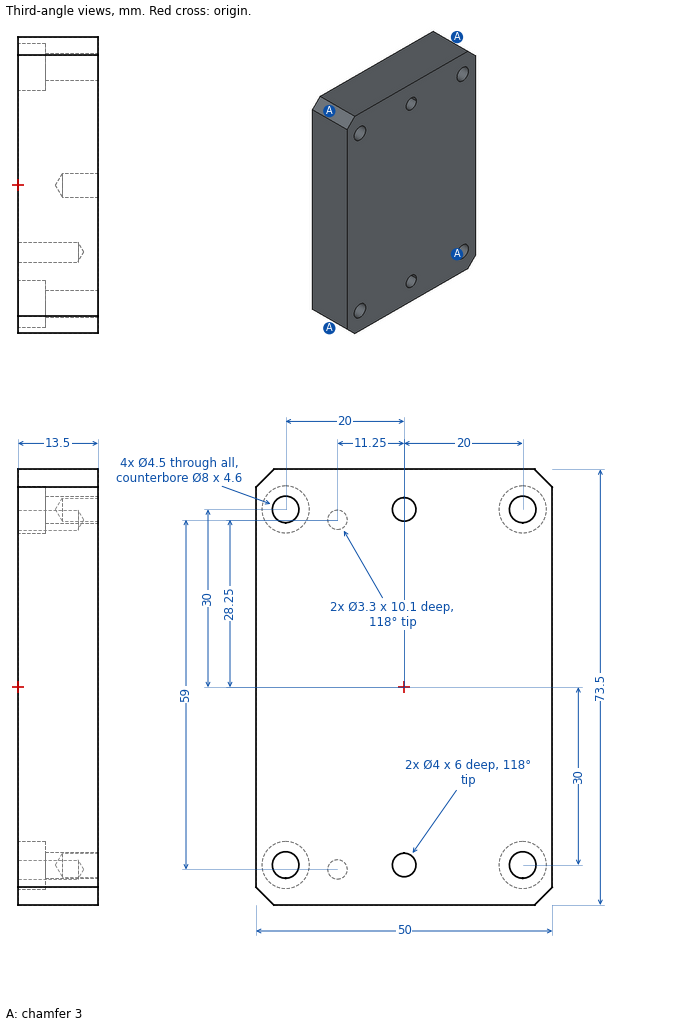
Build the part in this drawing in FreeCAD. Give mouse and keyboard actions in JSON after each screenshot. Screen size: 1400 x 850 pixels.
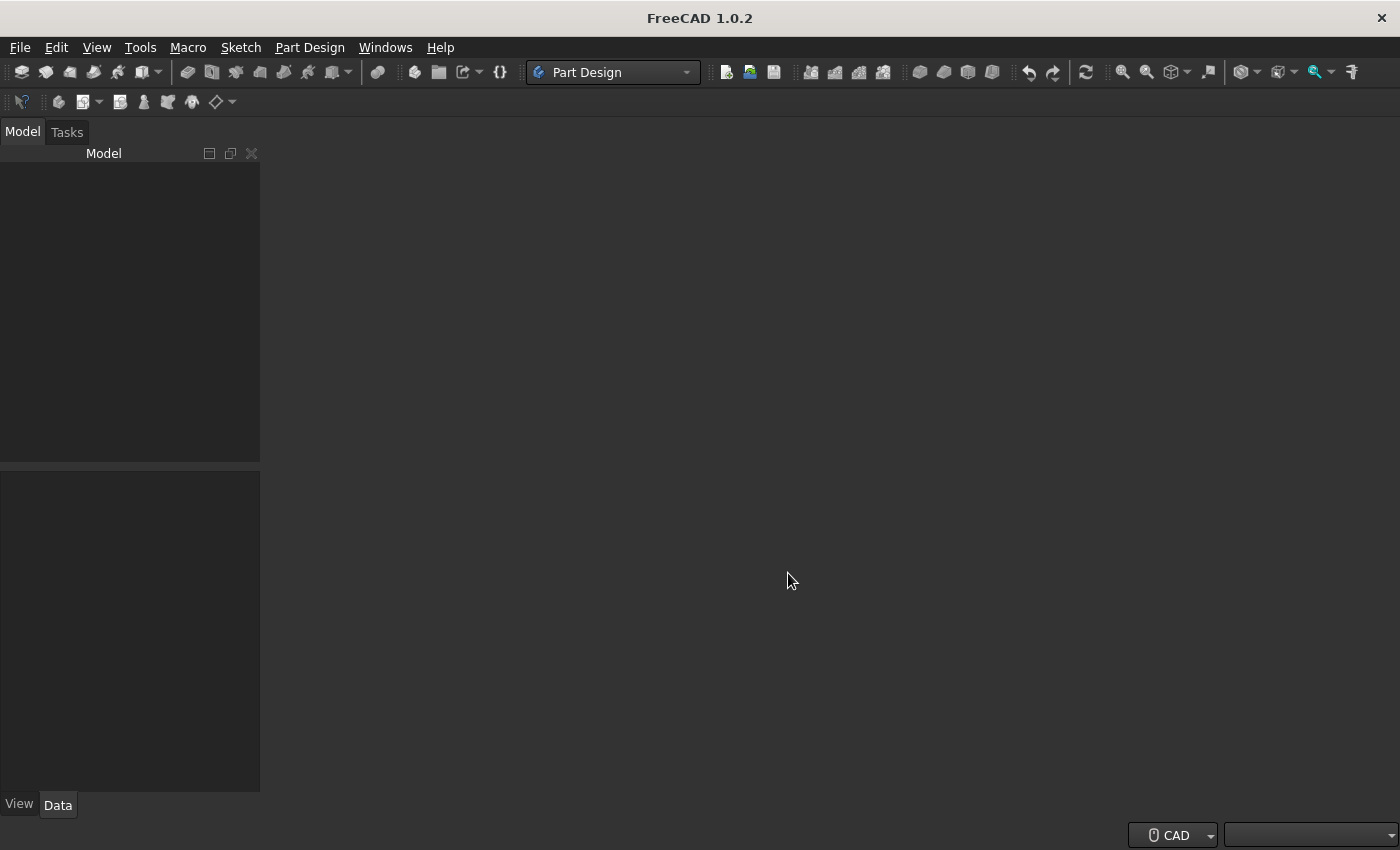
{"action": "left_click", "coordinate": [726, 72]}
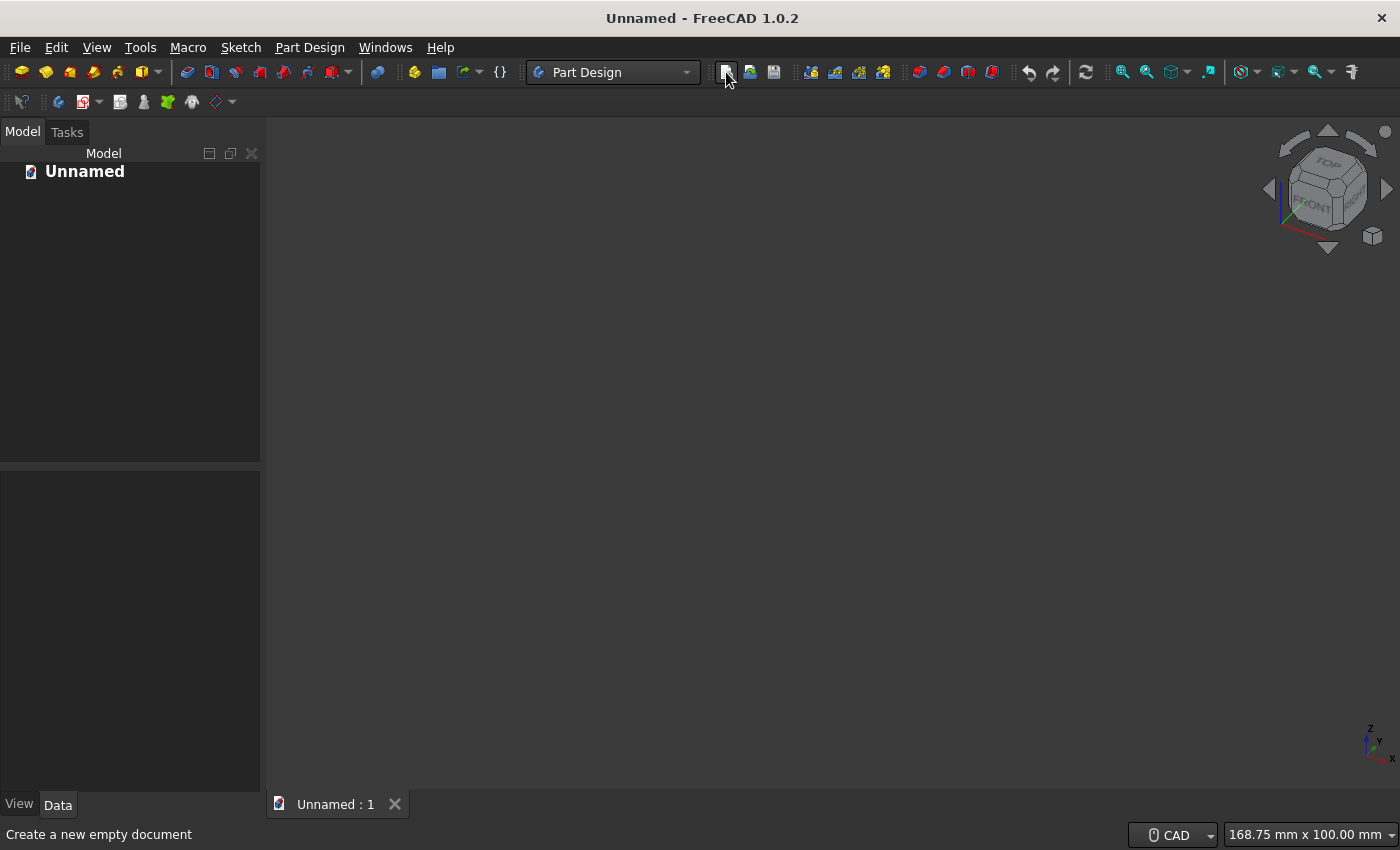
{"action": "left_click", "coordinate": [84, 102]}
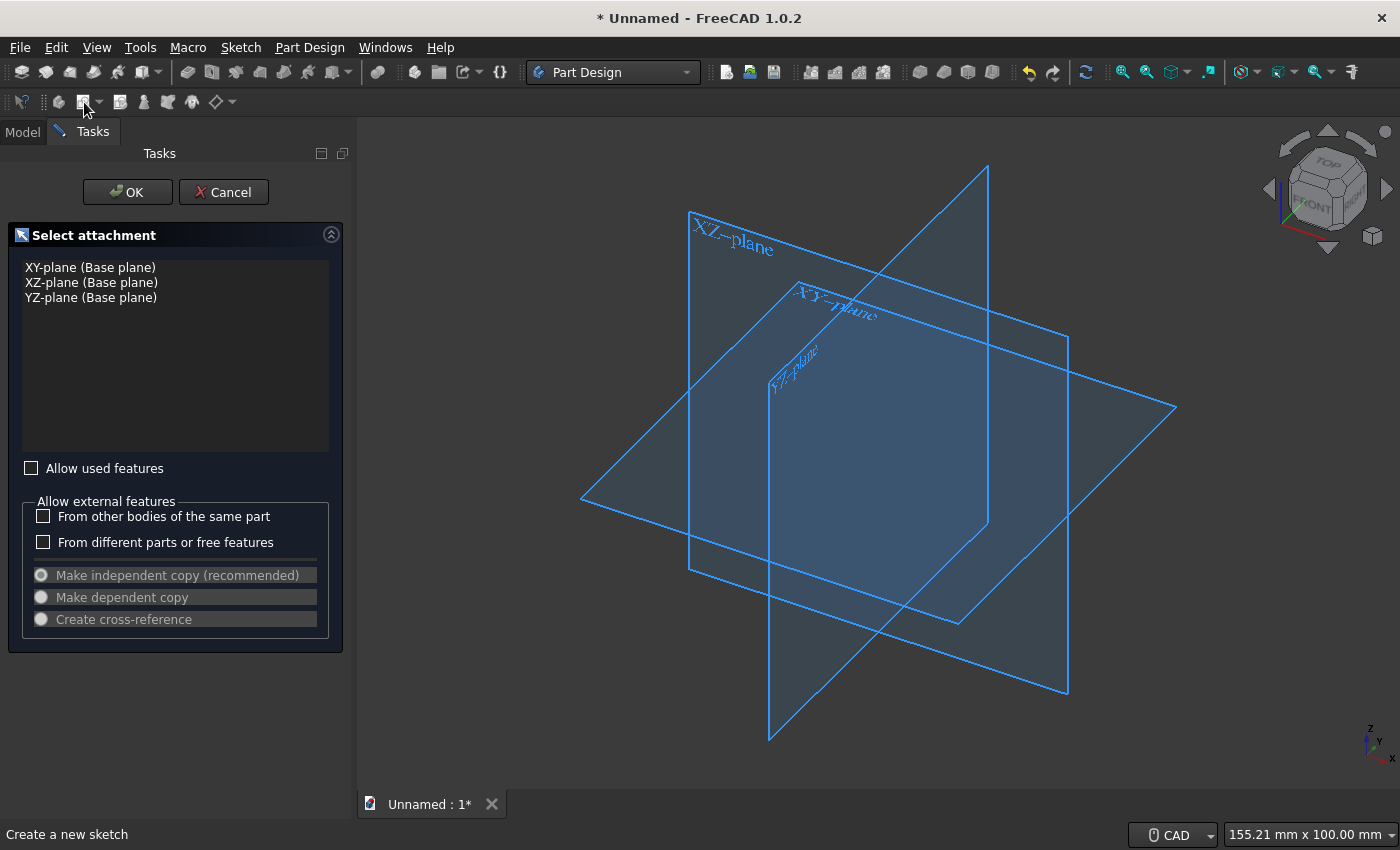
{"action": "left_click", "coordinate": [82, 298]}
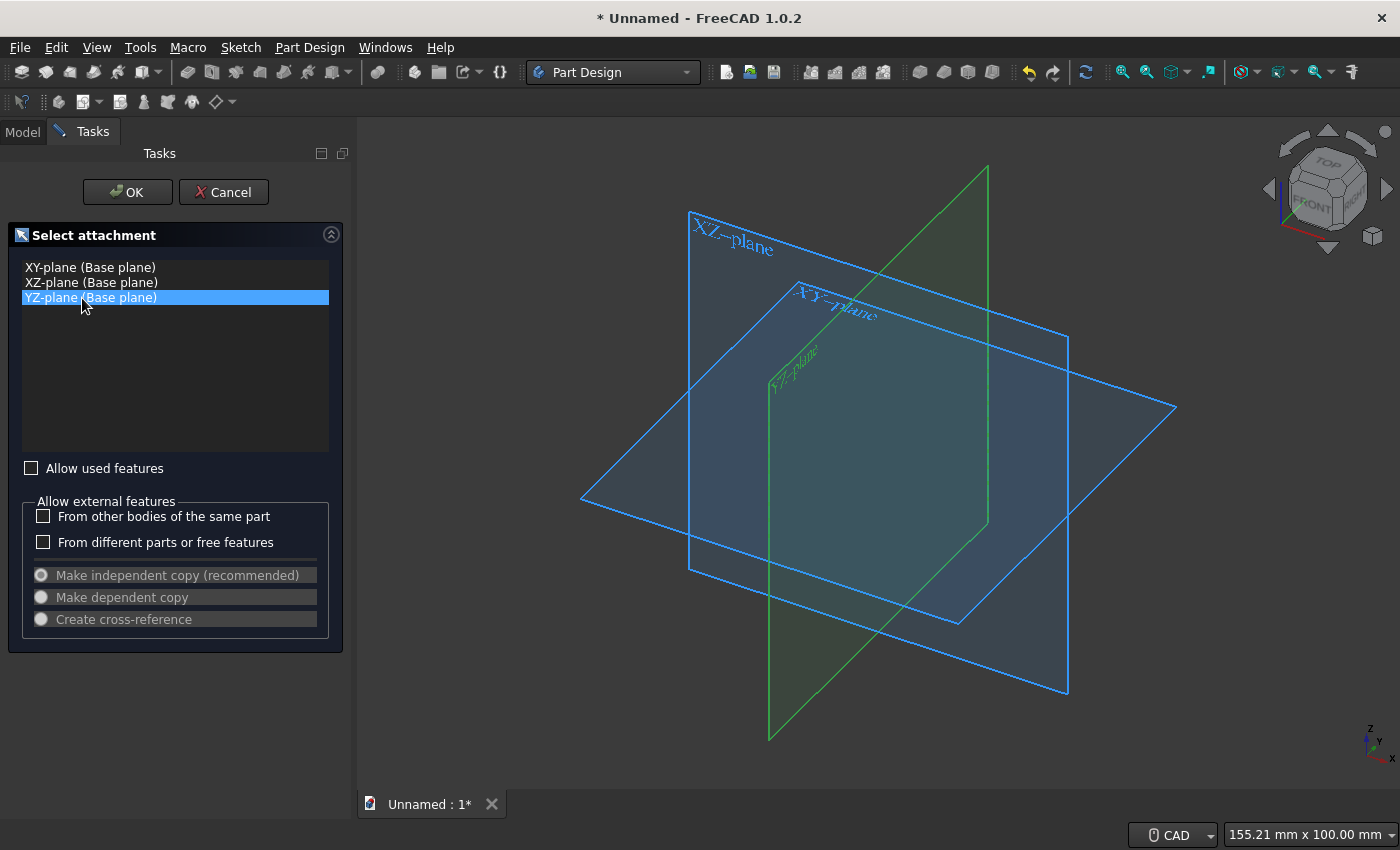
{"action": "left_click", "coordinate": [128, 192]}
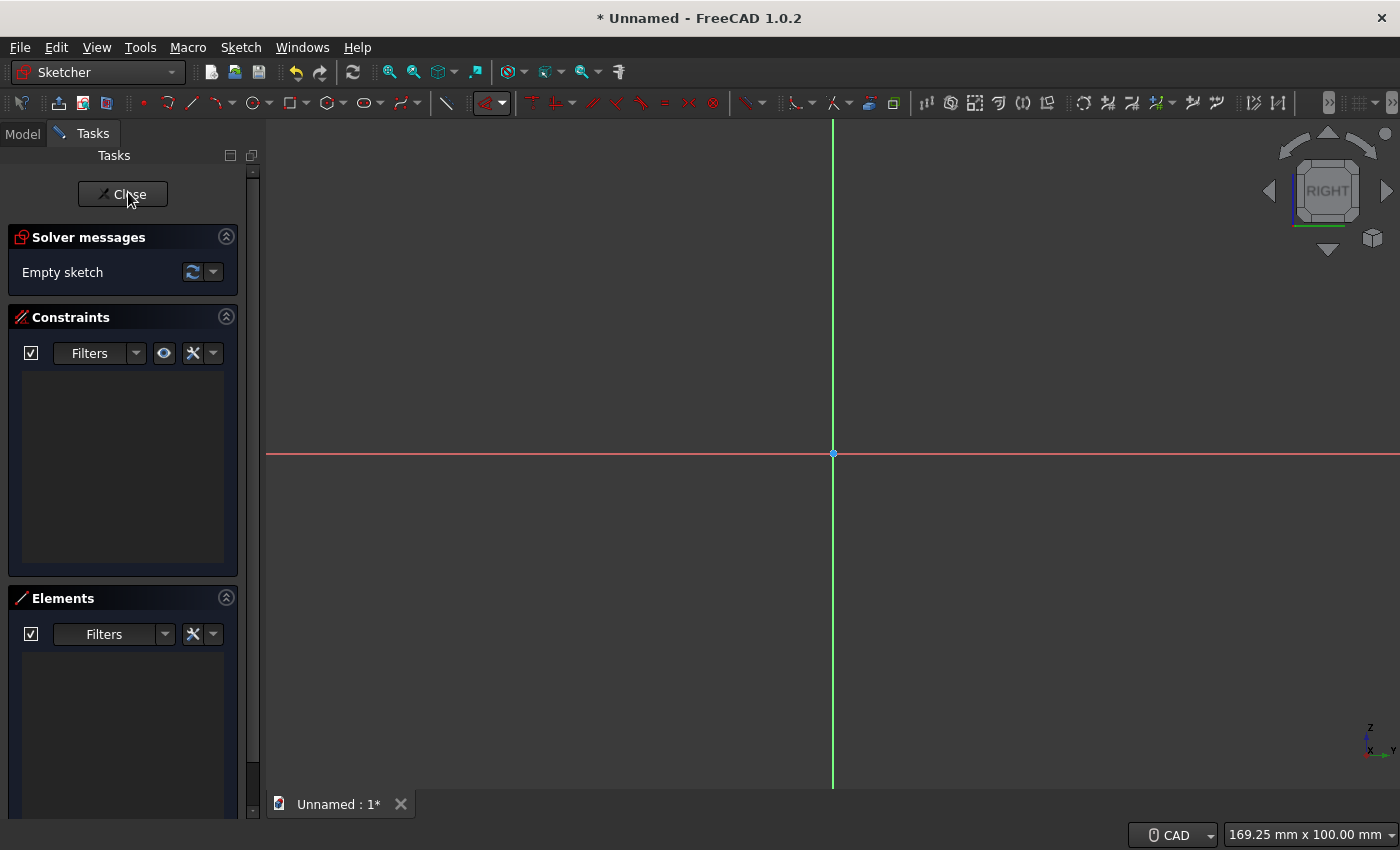
{"action": "key", "text": "g v"}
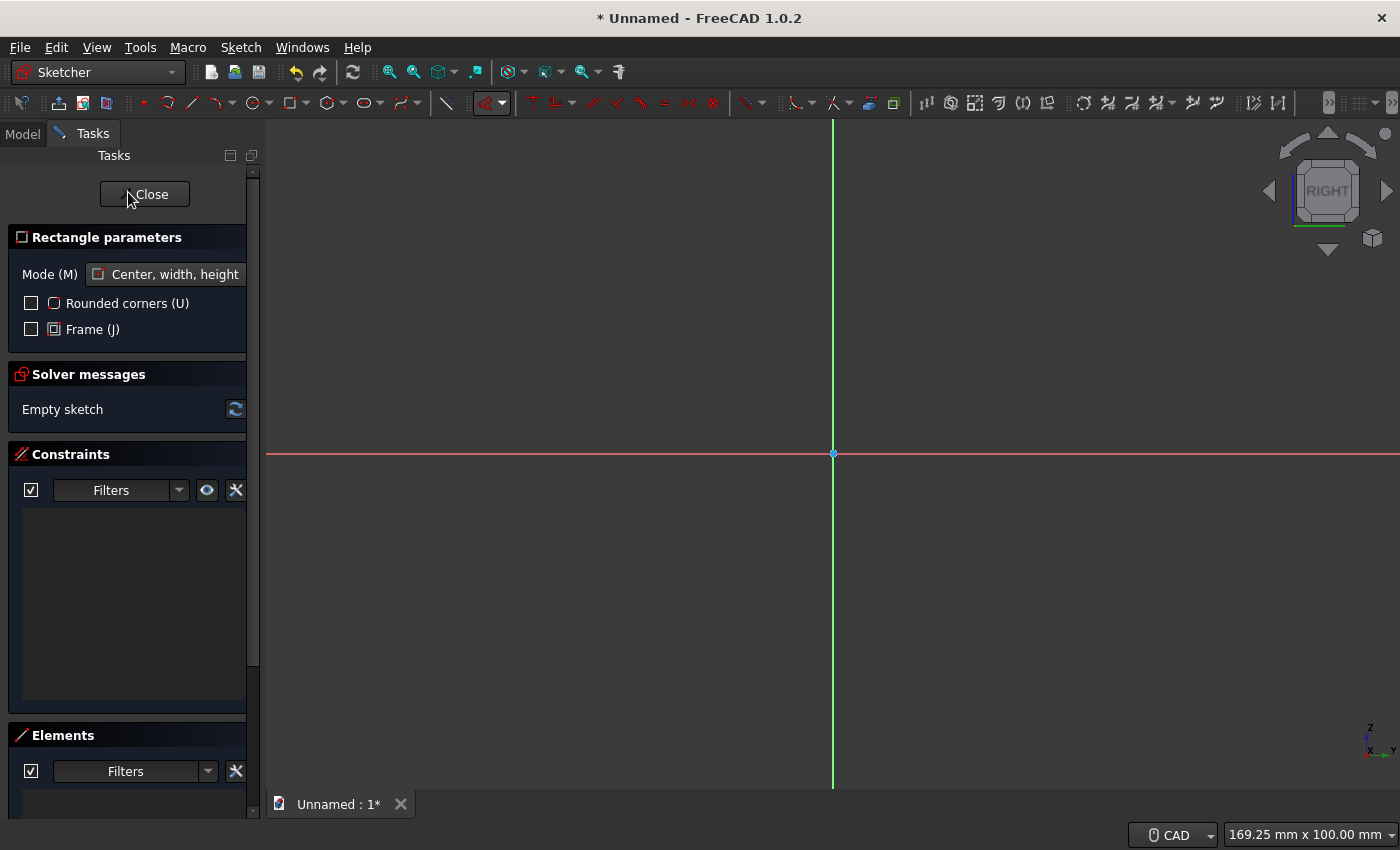
{"action": "left_click", "coordinate": [833, 454]}
{"action": "mouse_move", "coordinate": [1000, 208]}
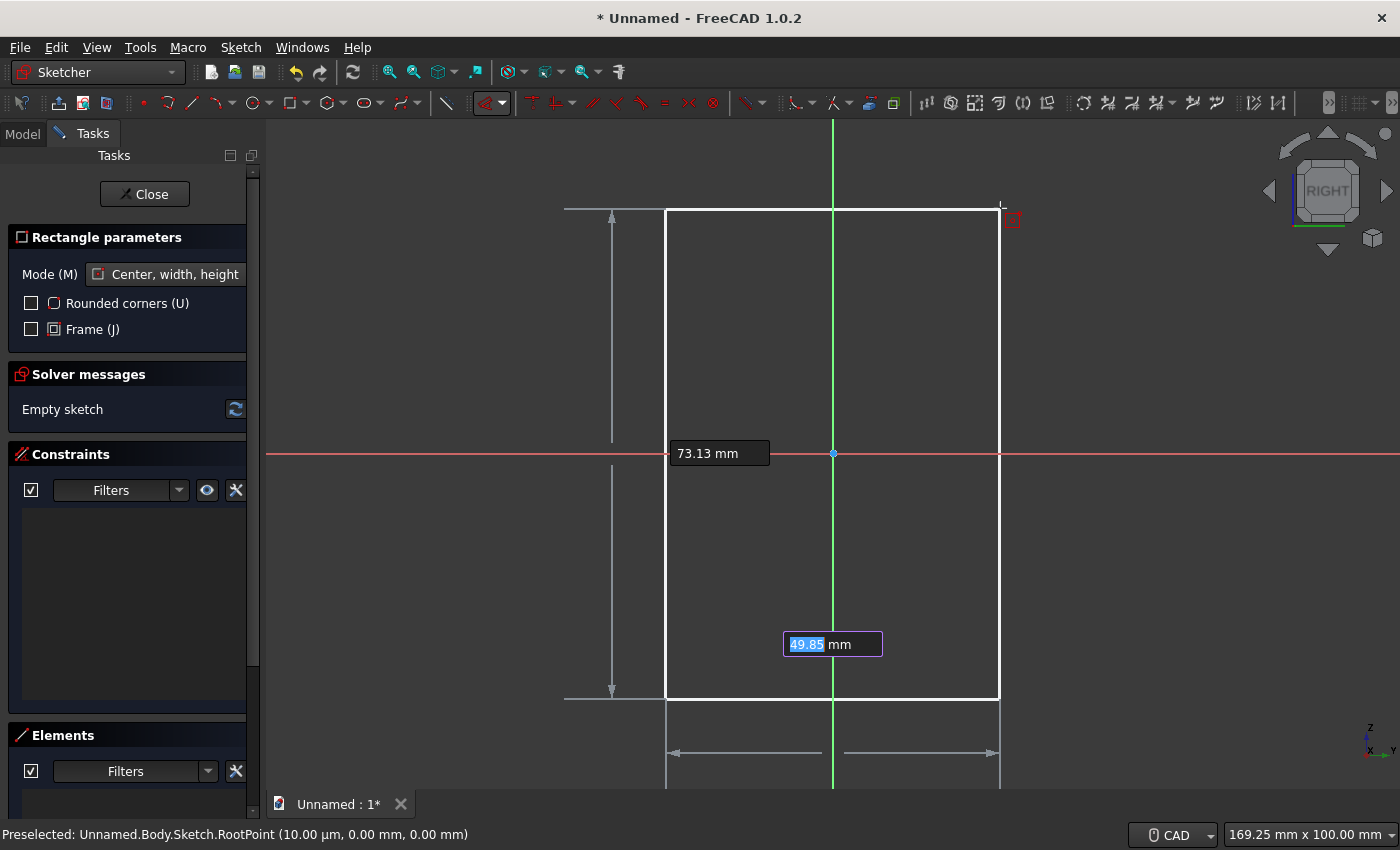
{"action": "type", "text": "50"}
{"action": "key", "text": "Tab"}
{"action": "type", "text": "73.5"}
{"action": "key", "text": "Return"}
{"action": "key", "text": "Escape"}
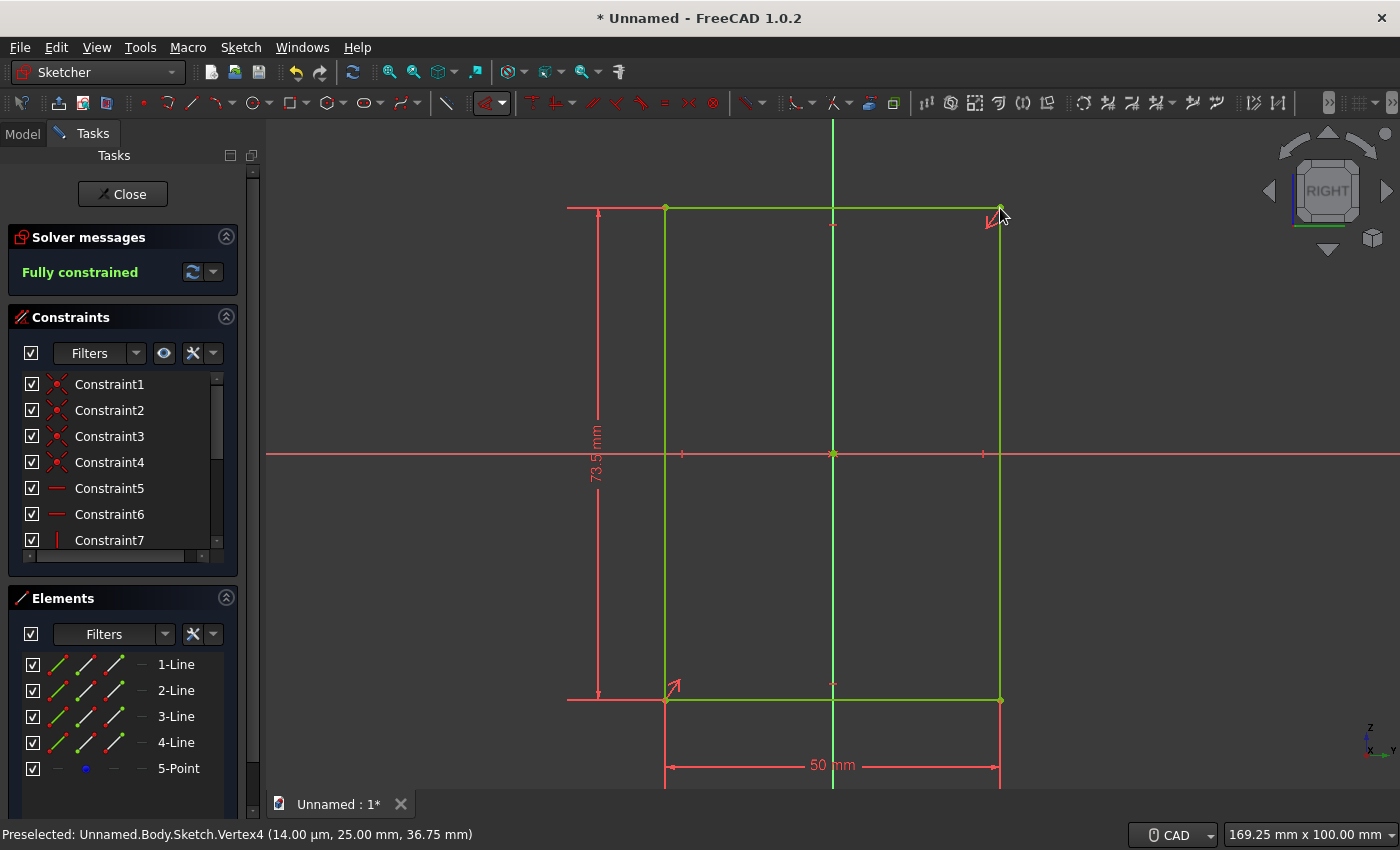
{"action": "left_click", "coordinate": [123, 194]}